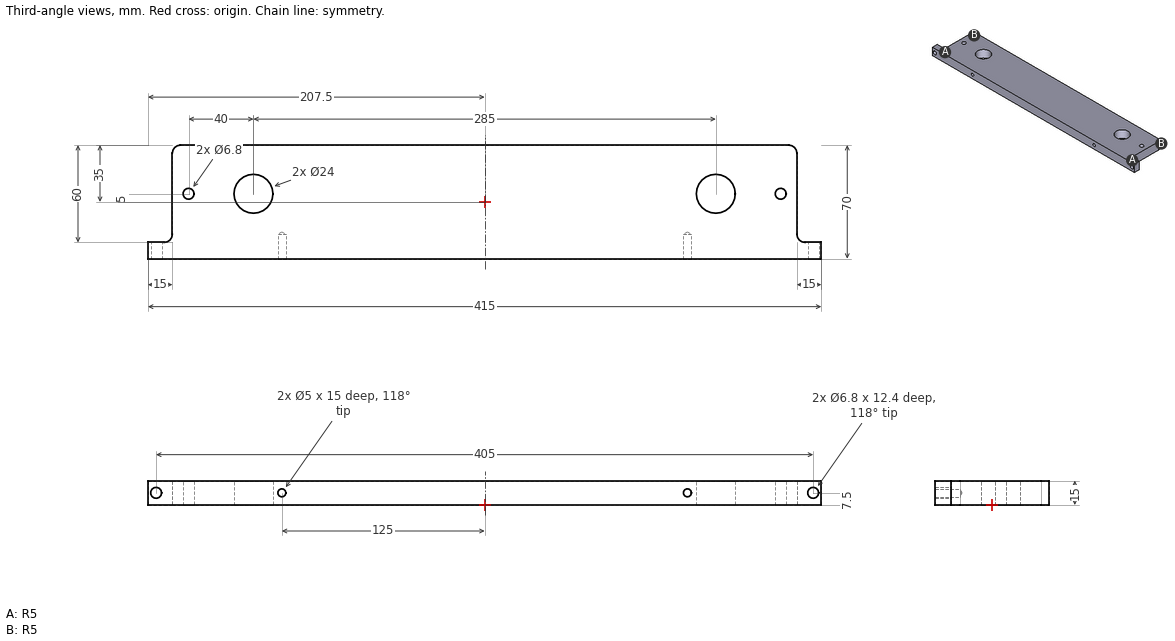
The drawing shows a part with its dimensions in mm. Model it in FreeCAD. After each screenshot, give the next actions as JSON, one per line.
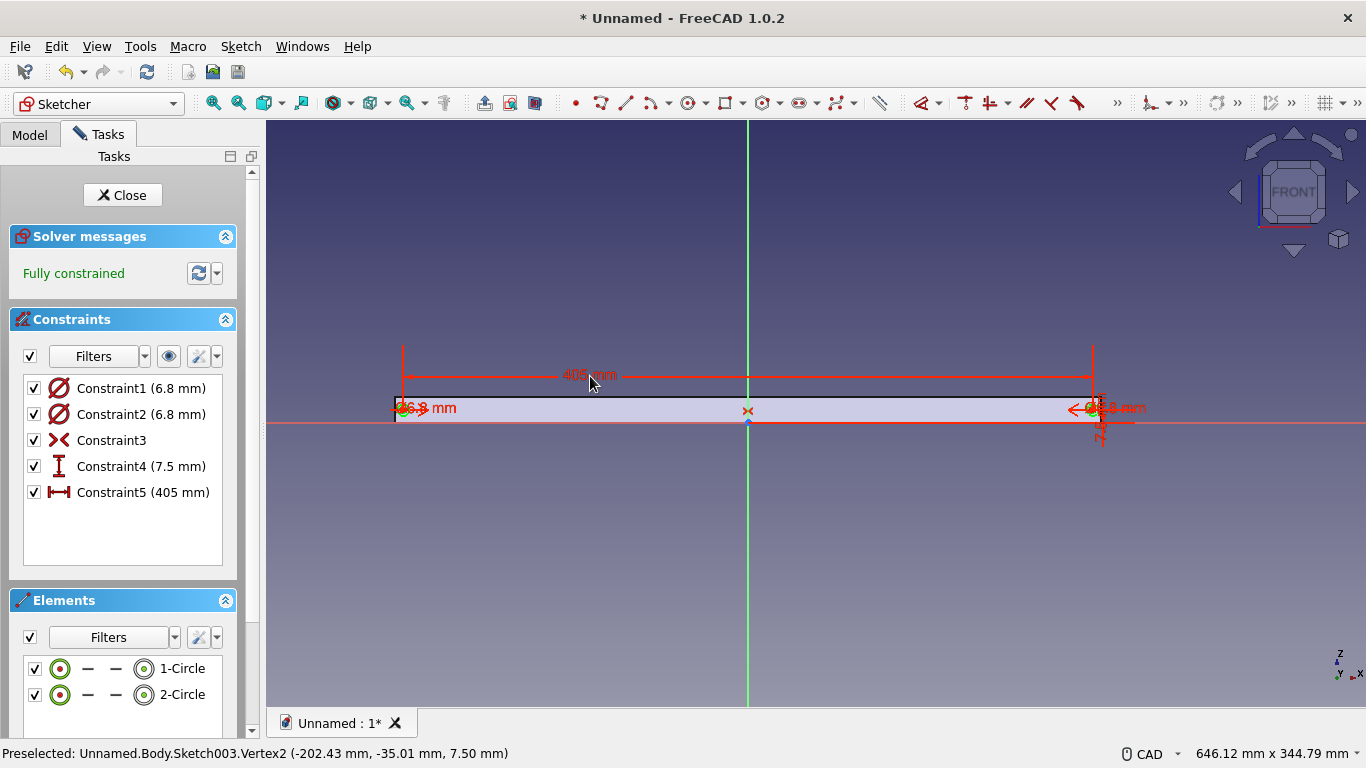
{"action": "left_click", "coordinate": [123, 195]}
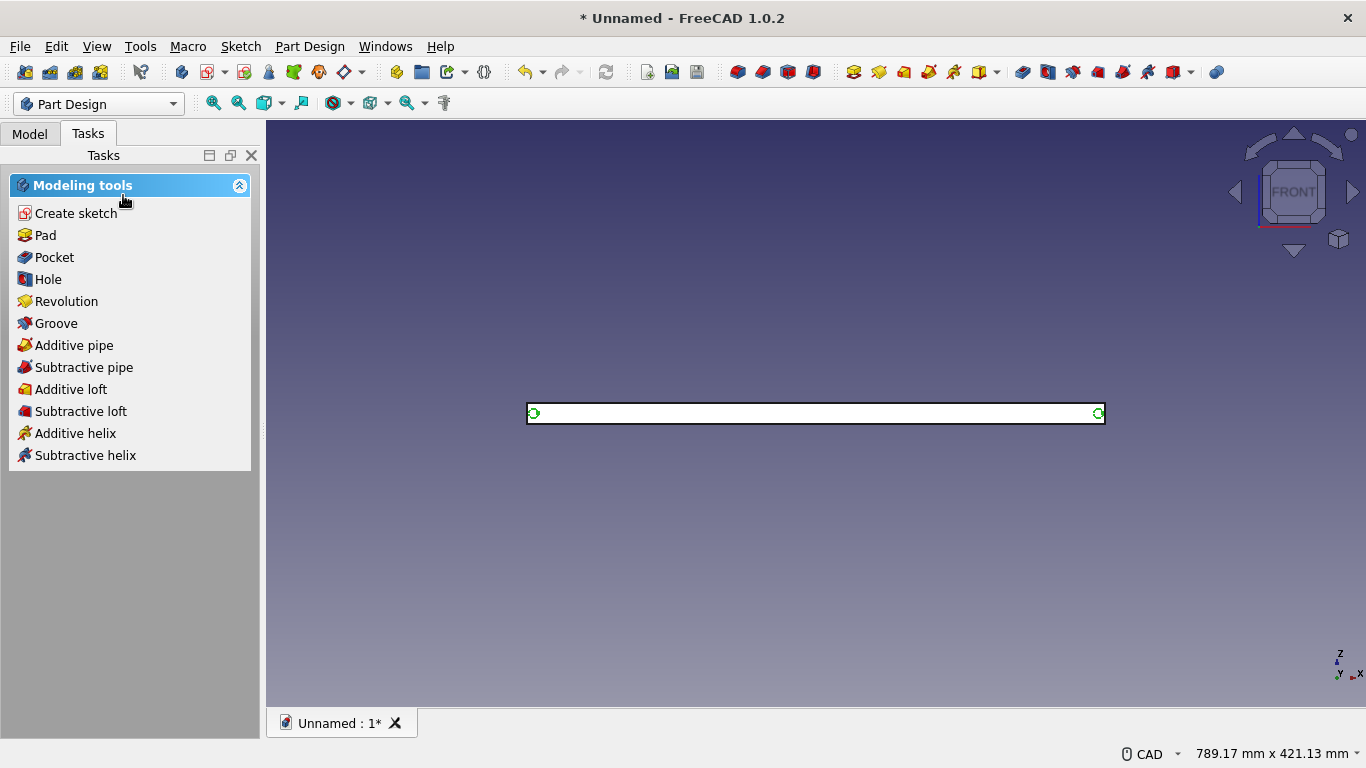
{"action": "left_click", "coordinate": [1048, 72]}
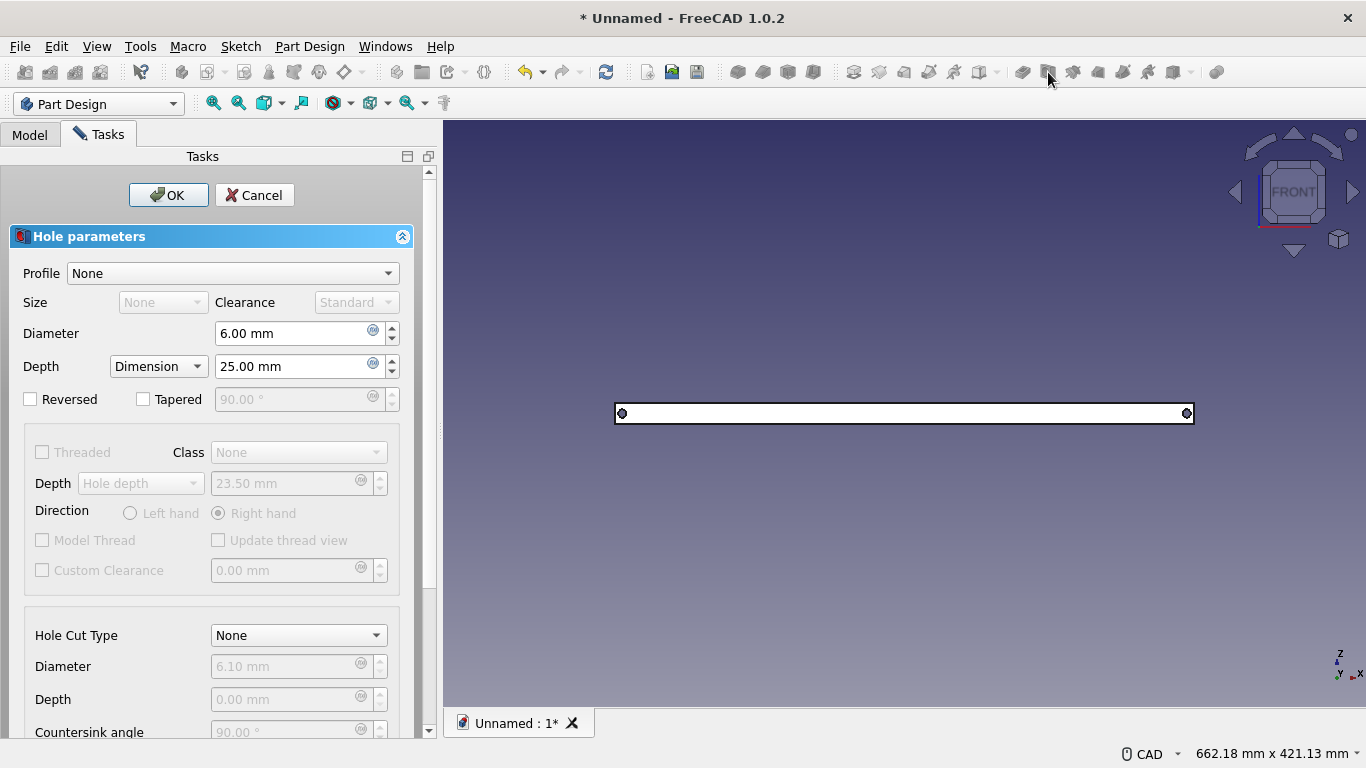
{"action": "triple_click", "coordinate": [300, 334]}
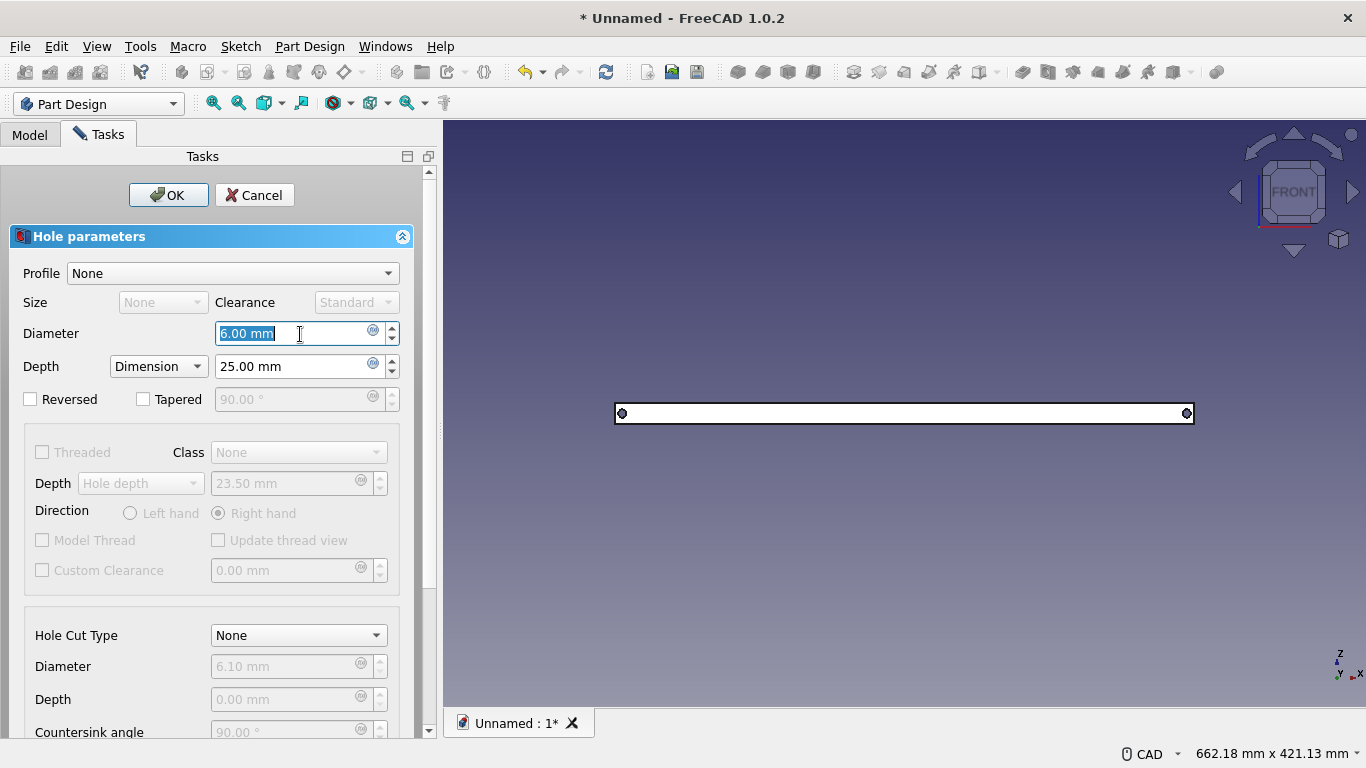
{"action": "type", "text": "6.8"}
{"action": "key", "text": "Tab"}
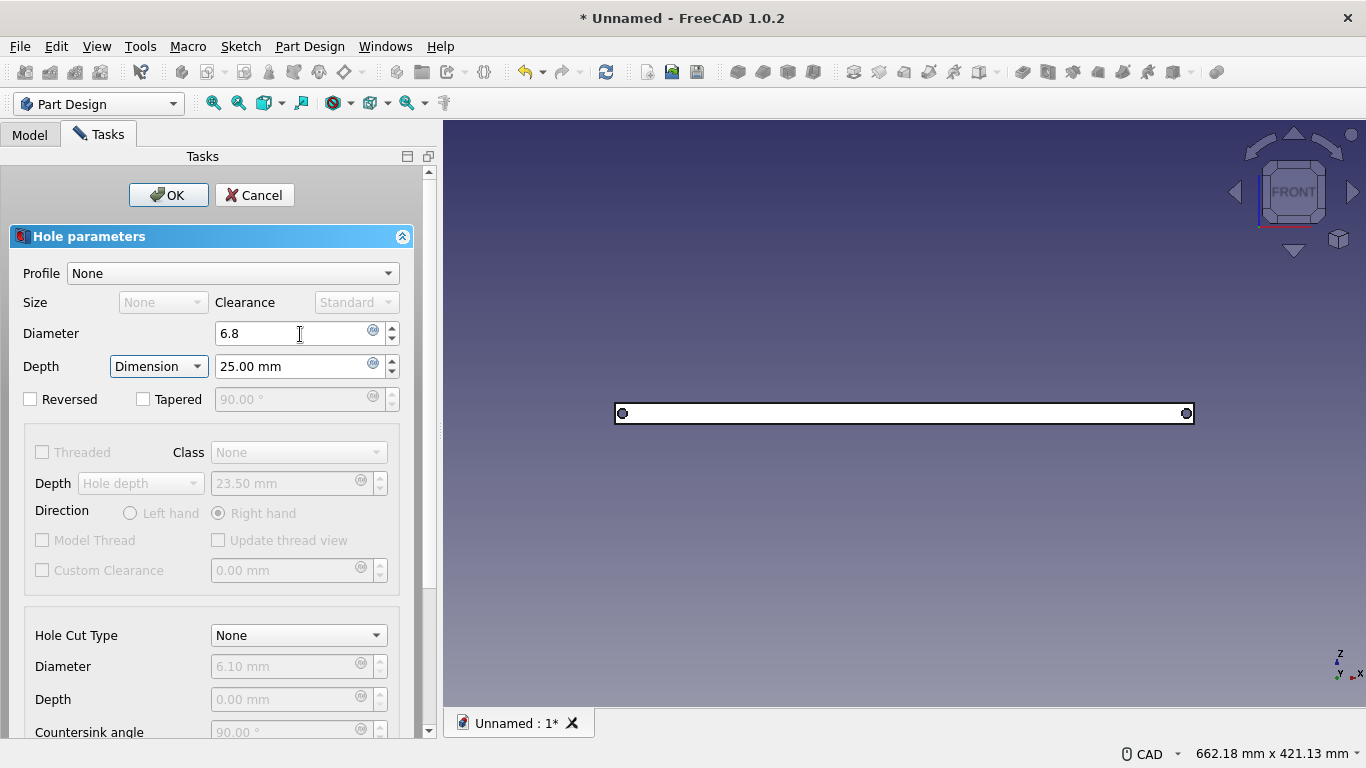
{"action": "triple_click", "coordinate": [300, 366]}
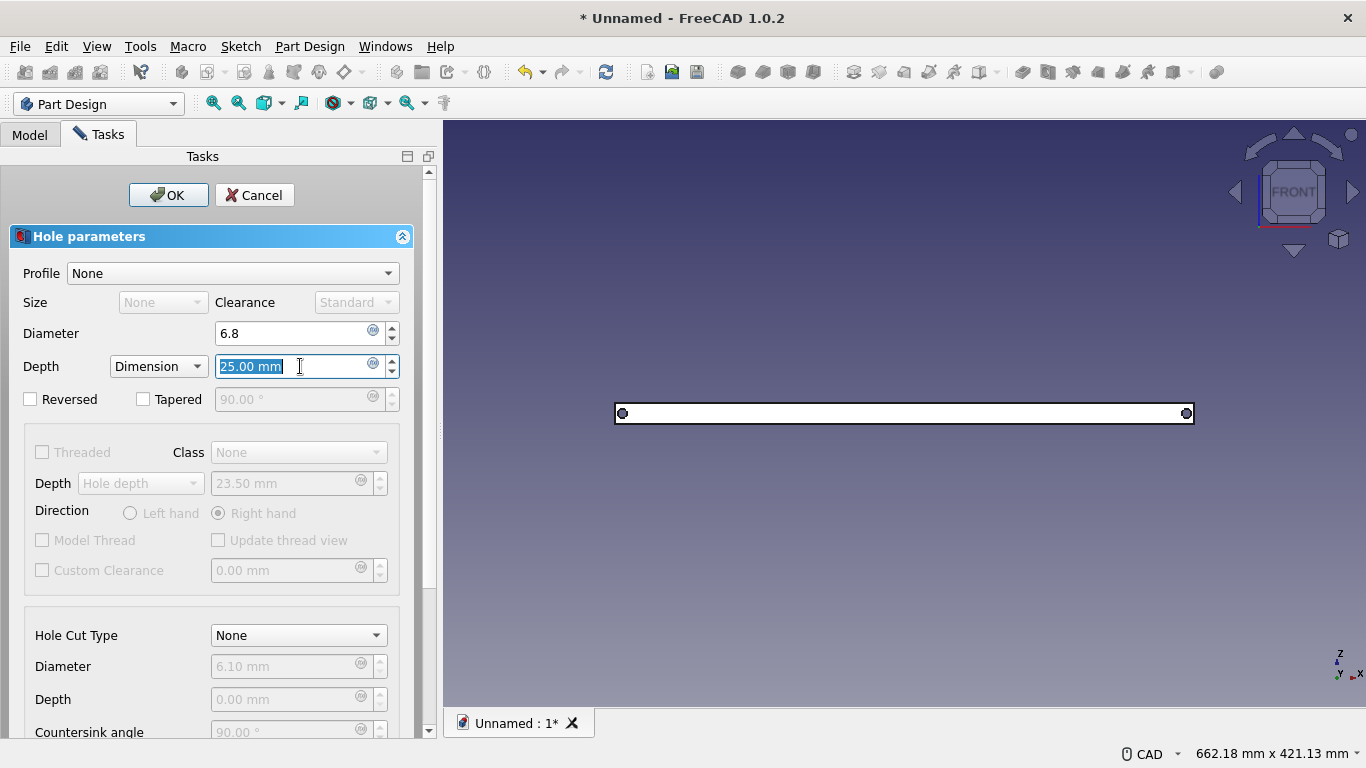
{"action": "type", "text": "12.4"}
{"action": "key", "text": "Tab"}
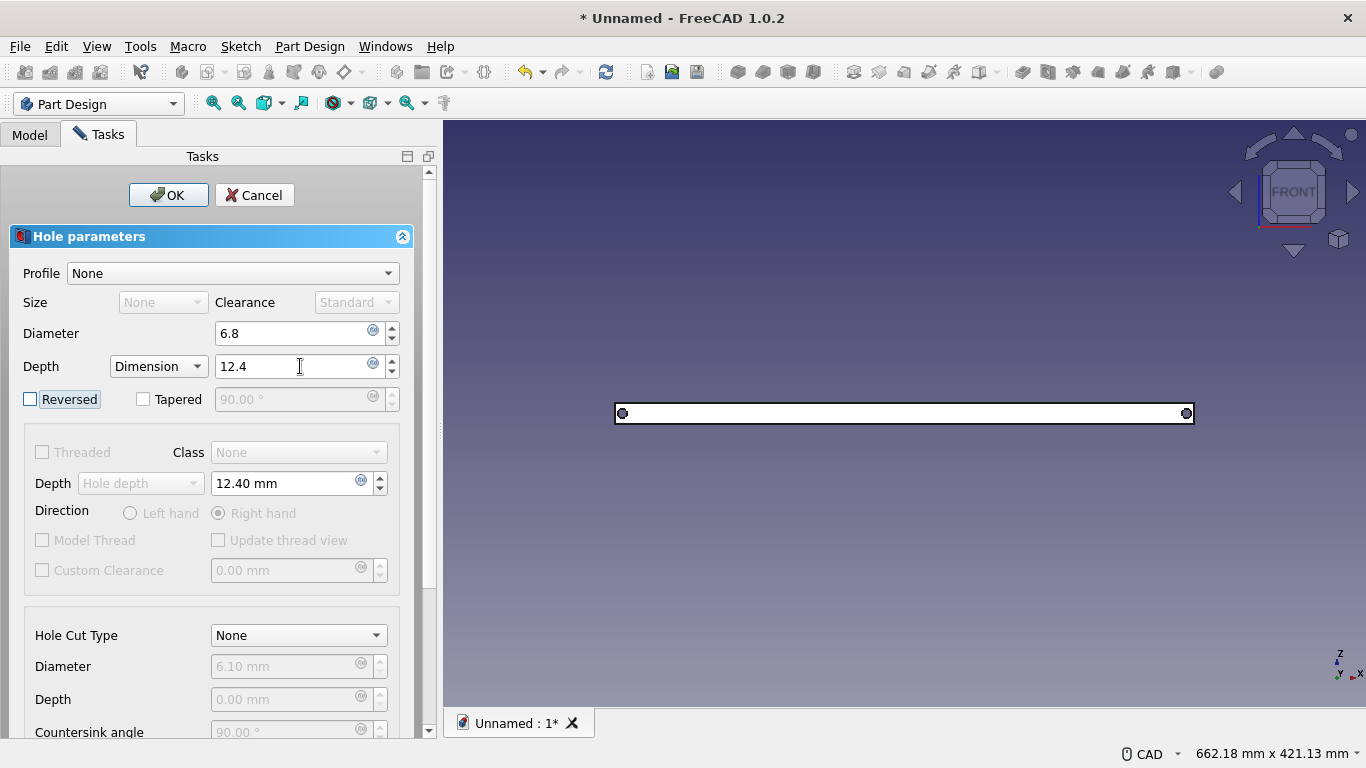
{"action": "left_click", "coordinate": [169, 195]}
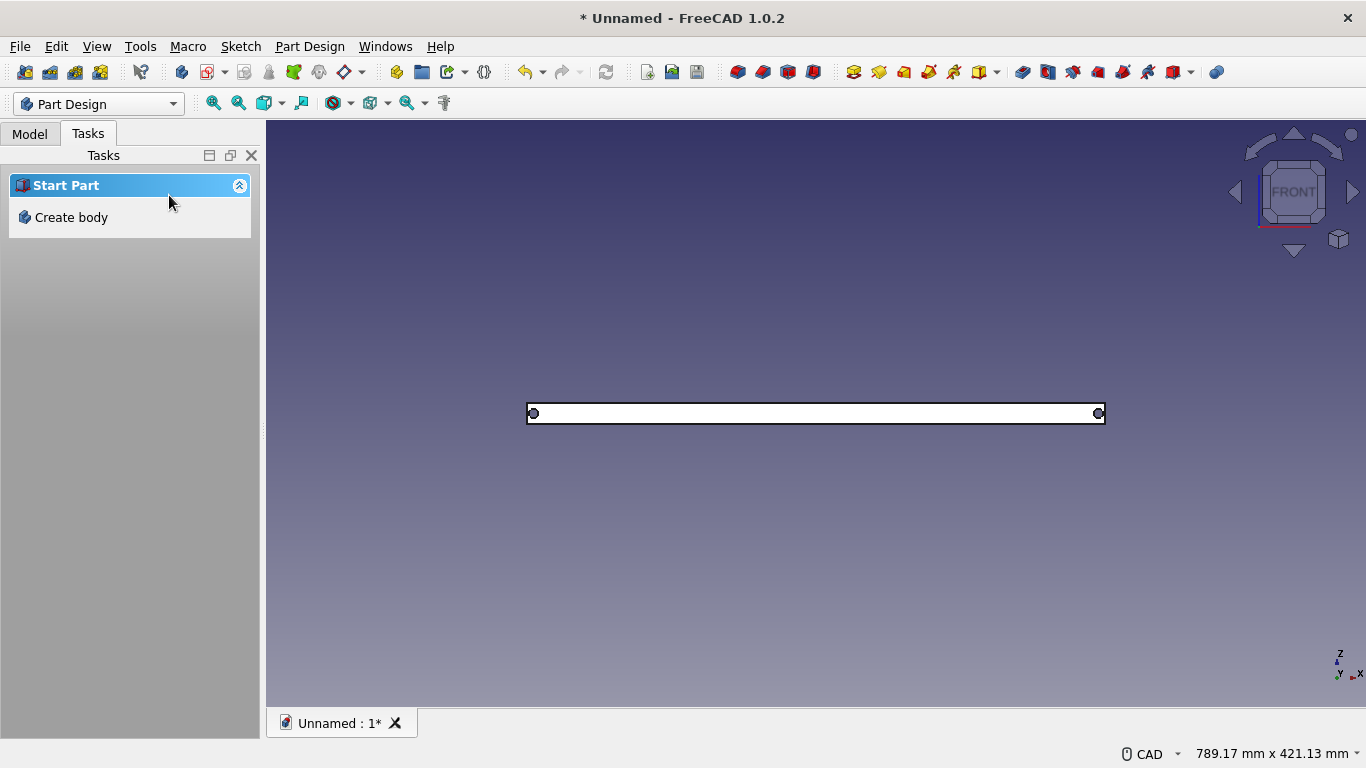
{"action": "scroll", "coordinate": [548, 412], "scroll_direction": "up", "scroll_amount": 4}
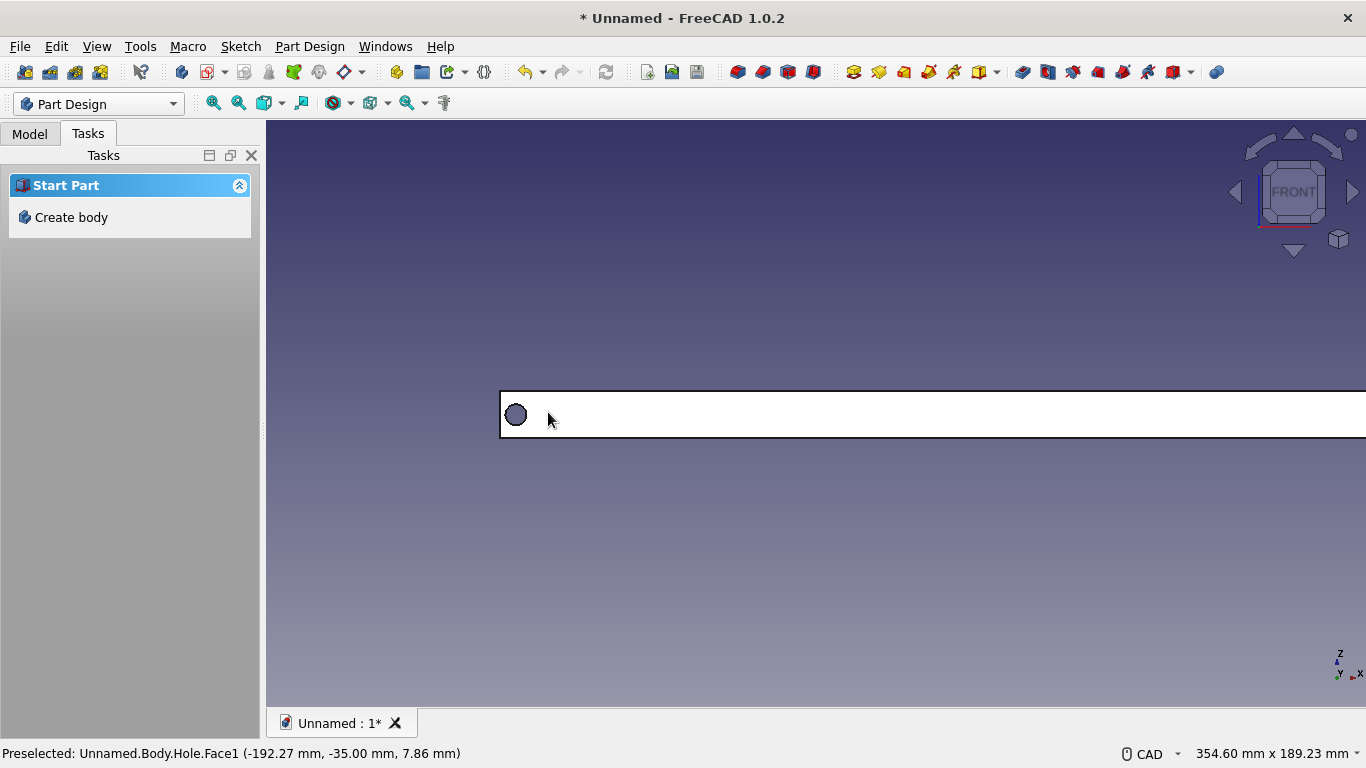
{"action": "left_click", "coordinate": [214, 104]}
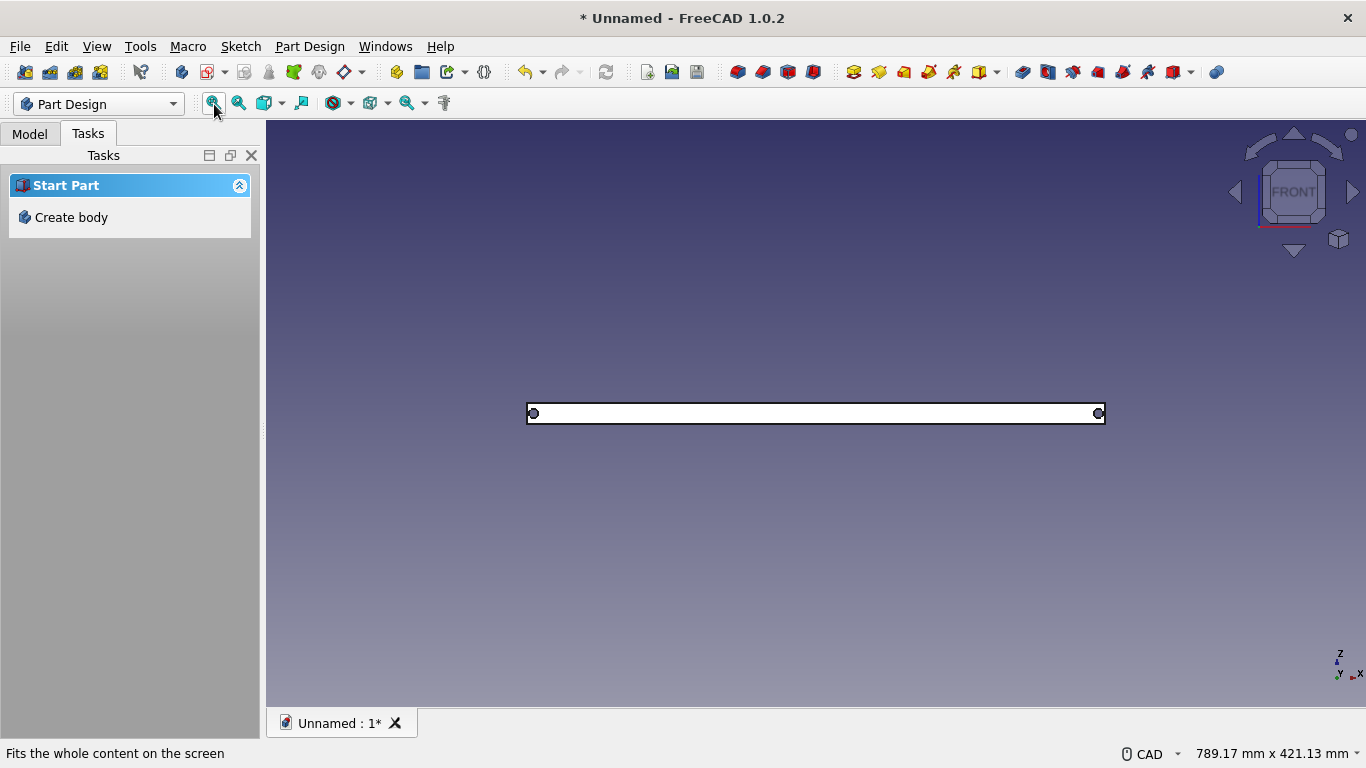
{"action": "key", "text": "0"}